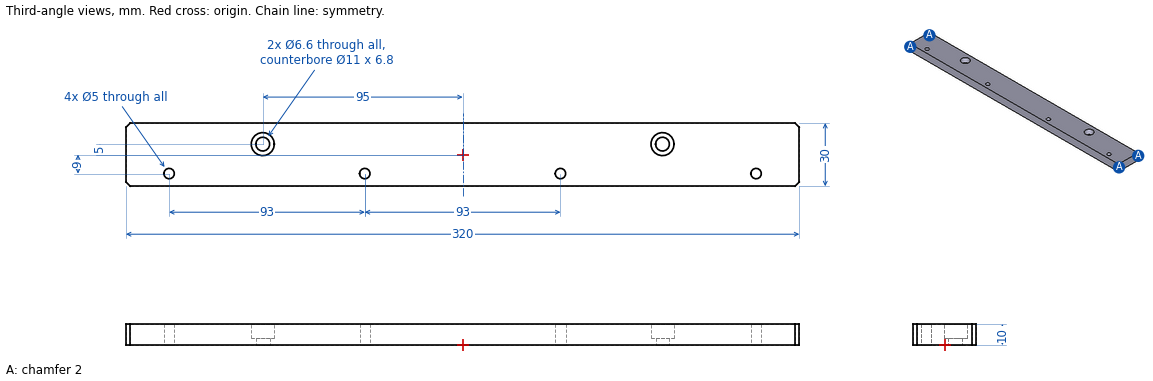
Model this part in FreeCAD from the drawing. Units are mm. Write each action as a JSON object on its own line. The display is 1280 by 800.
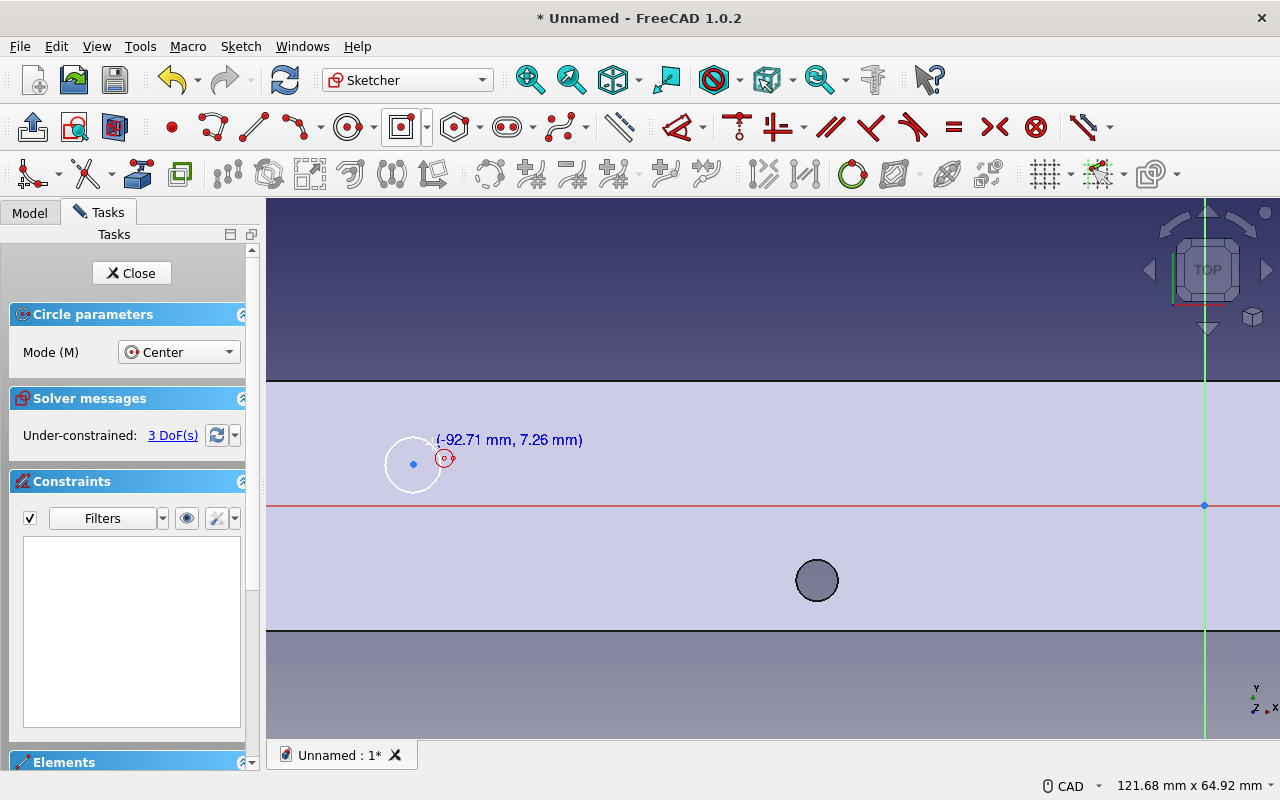
{"action": "scroll", "coordinate": [413, 467], "scroll_direction": "down", "scroll_amount": 5}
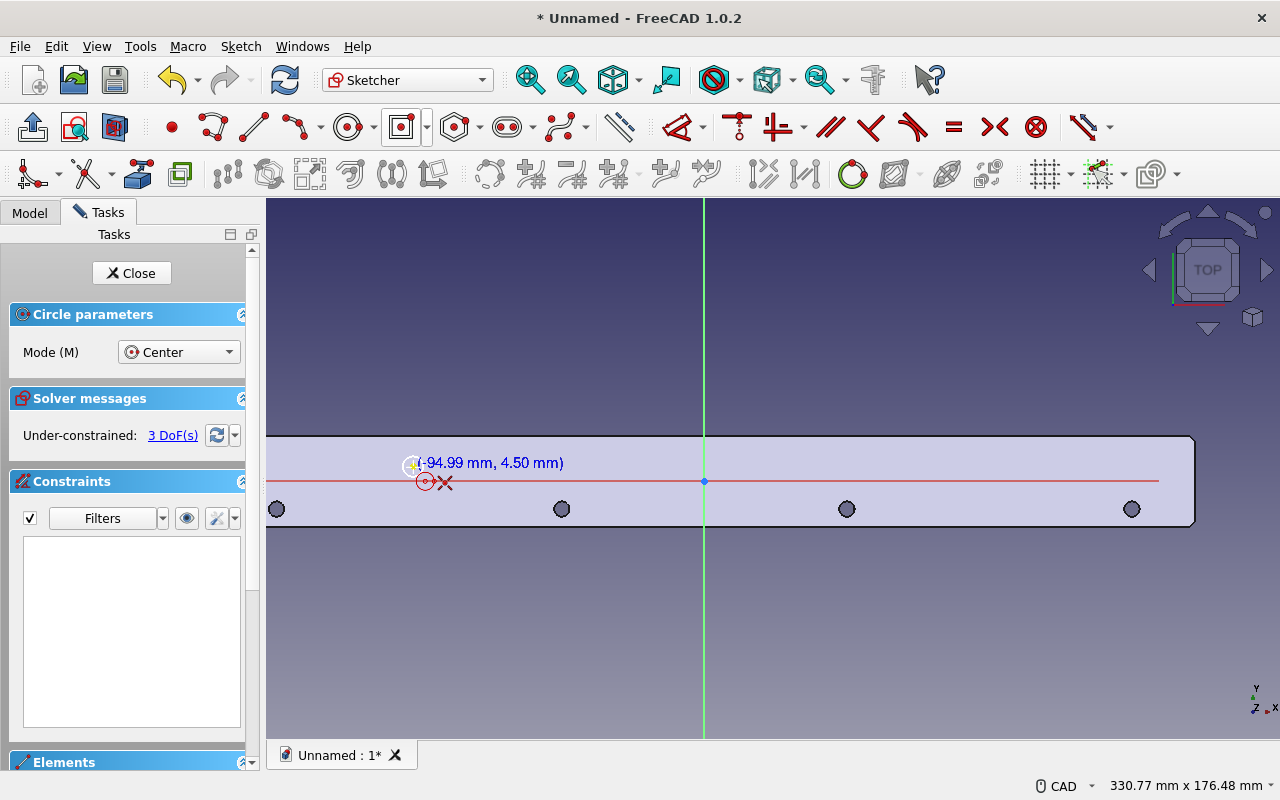
{"action": "scroll", "coordinate": [996, 466], "scroll_direction": "up", "scroll_amount": 5}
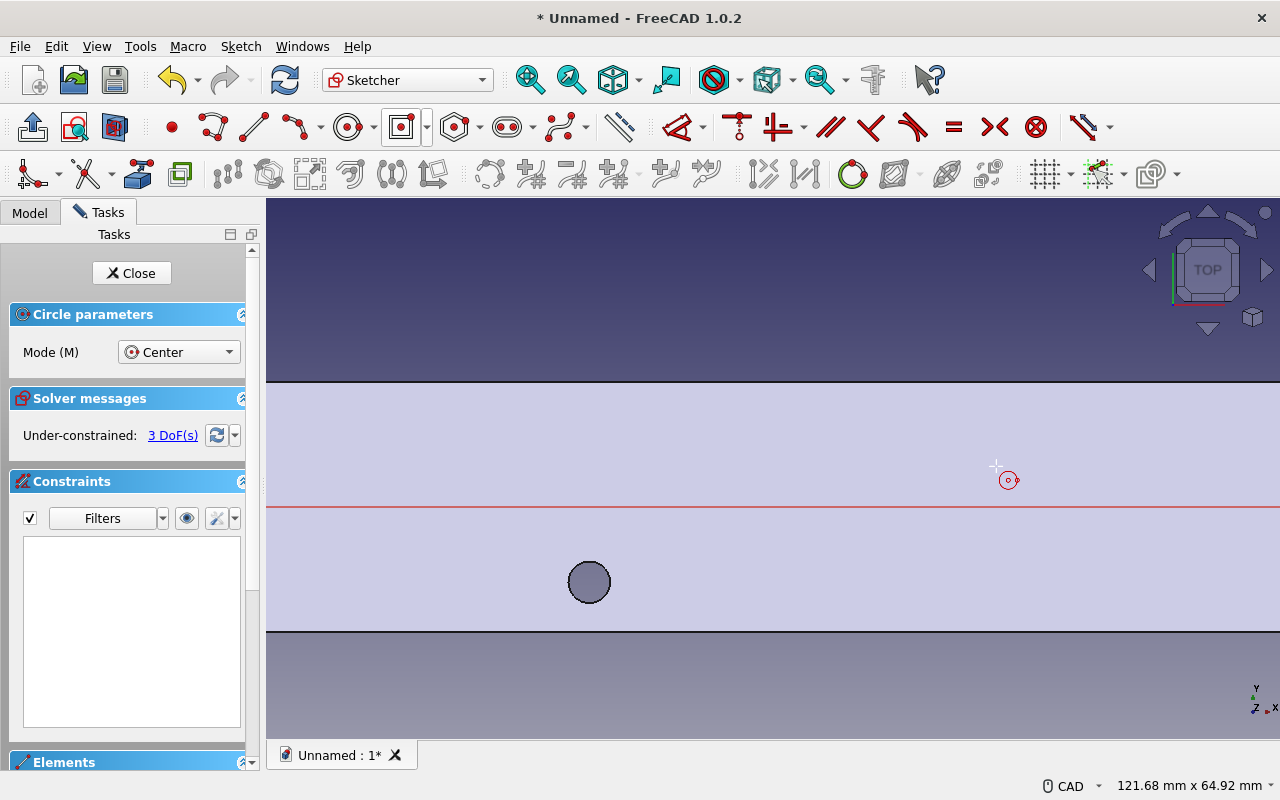
{"action": "left_click", "coordinate": [993, 466]}
{"action": "left_click", "coordinate": [1013, 446]}
{"action": "key", "text": "Escape"}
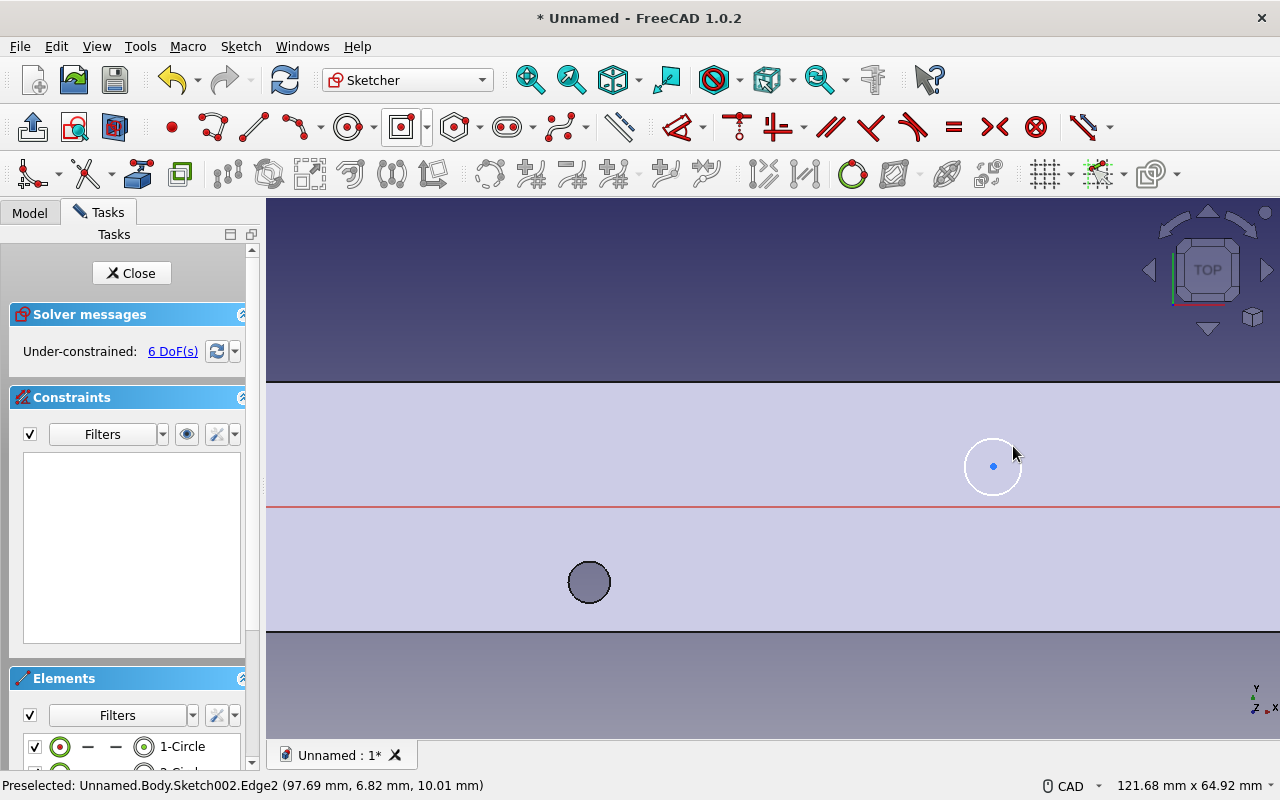
{"action": "scroll", "coordinate": [997, 466], "scroll_direction": "down", "scroll_amount": 5}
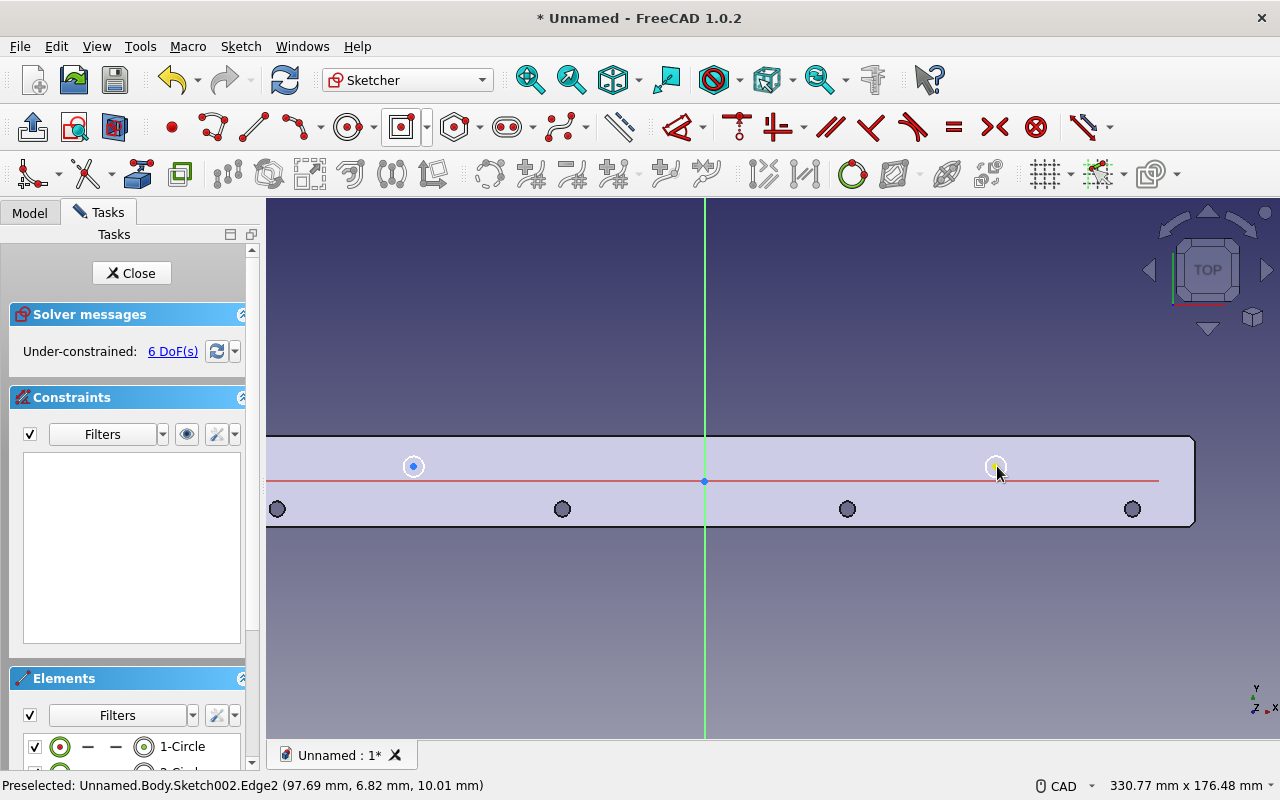
{"action": "scroll", "coordinate": [421, 459], "scroll_direction": "up", "scroll_amount": 2}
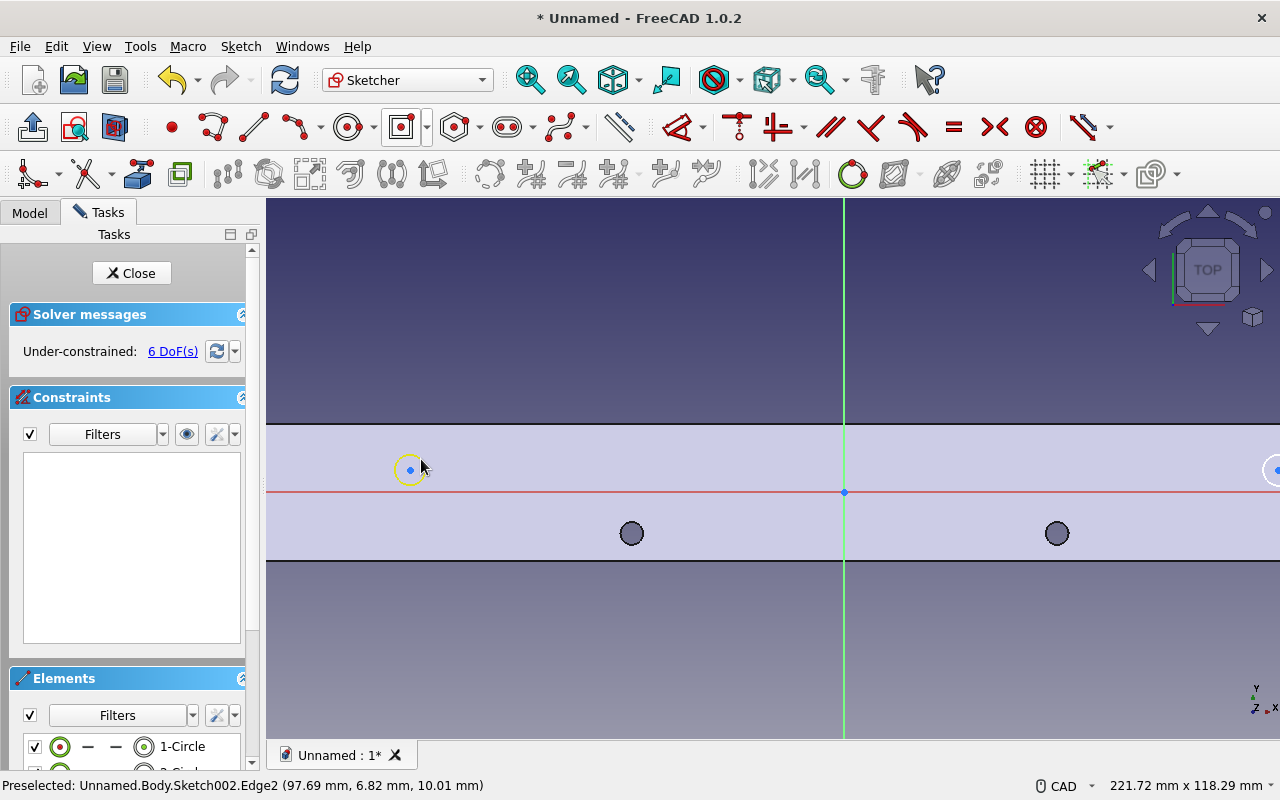
{"action": "left_click", "coordinate": [421, 459]}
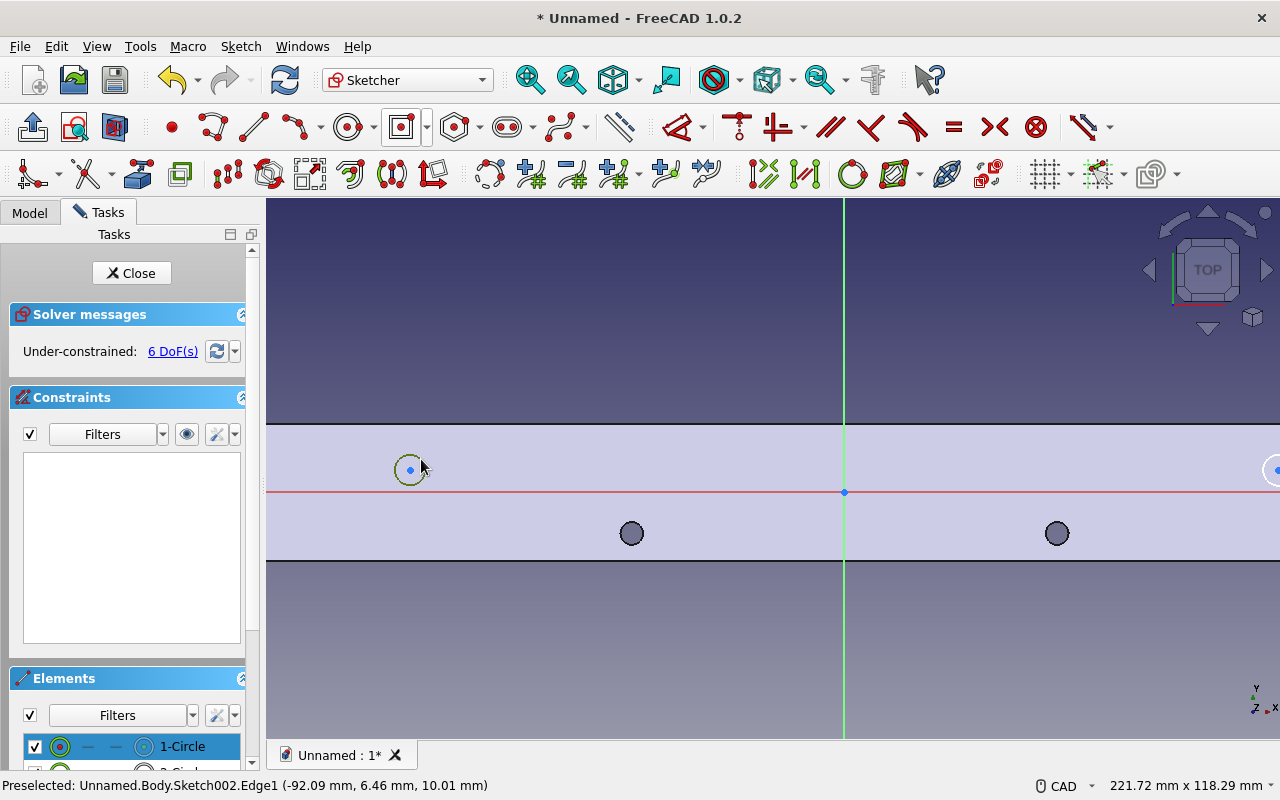
{"action": "scroll", "coordinate": [420, 459], "scroll_direction": "down", "scroll_amount": 2}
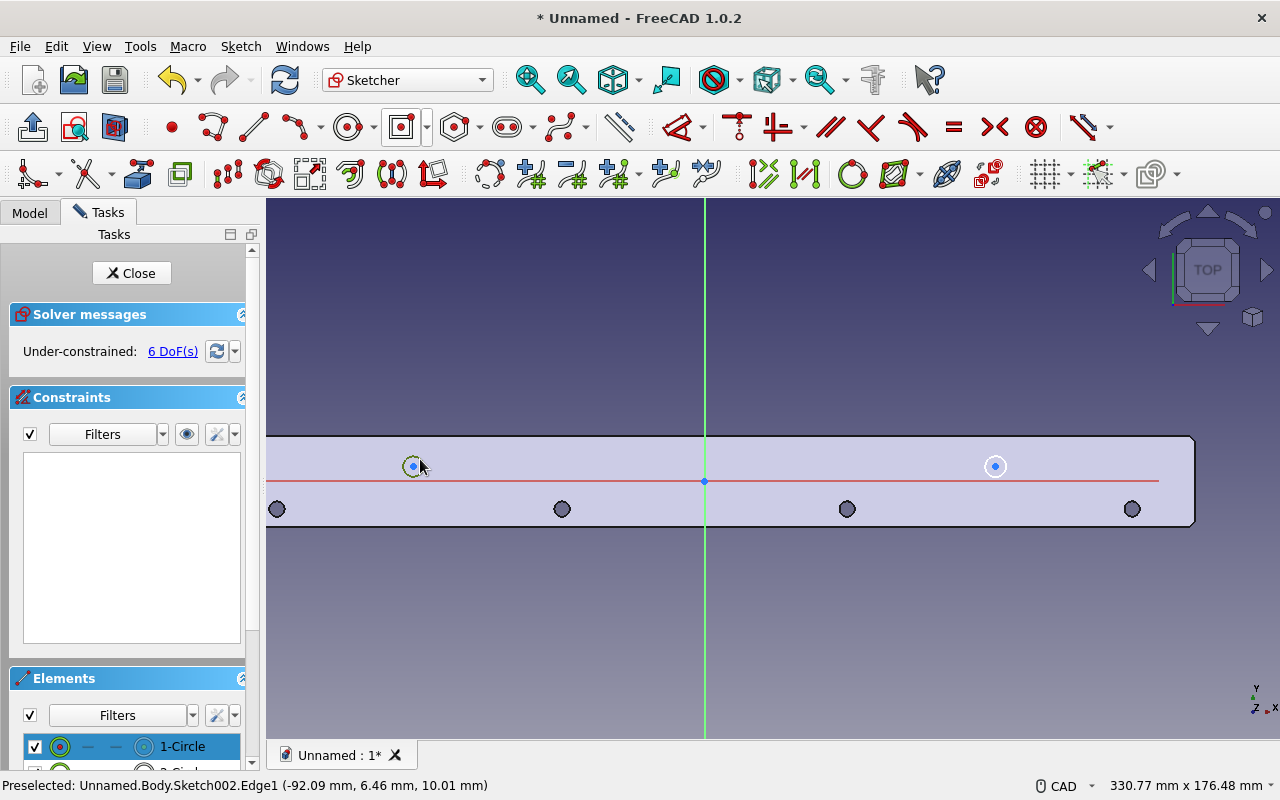
{"action": "scroll", "coordinate": [1003, 459], "scroll_direction": "up", "scroll_amount": 2}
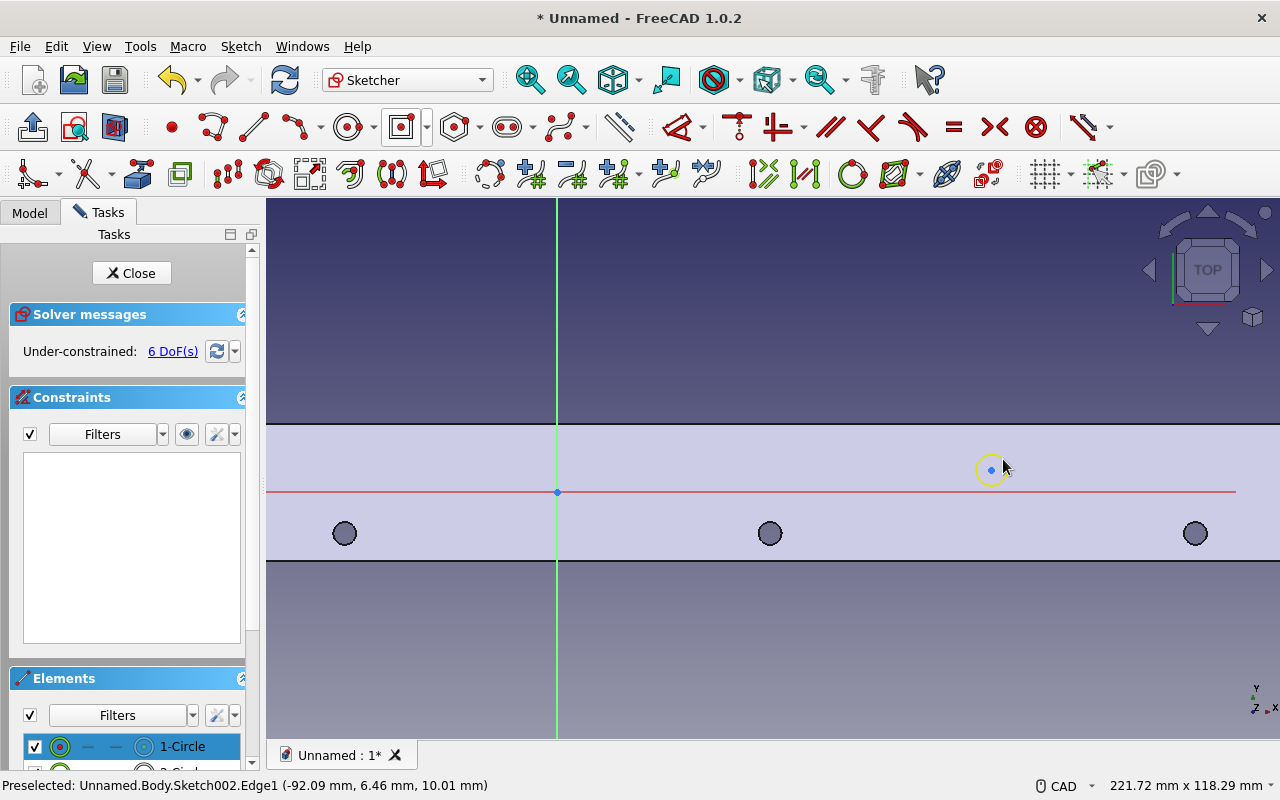
{"action": "left_click", "coordinate": [1003, 459]}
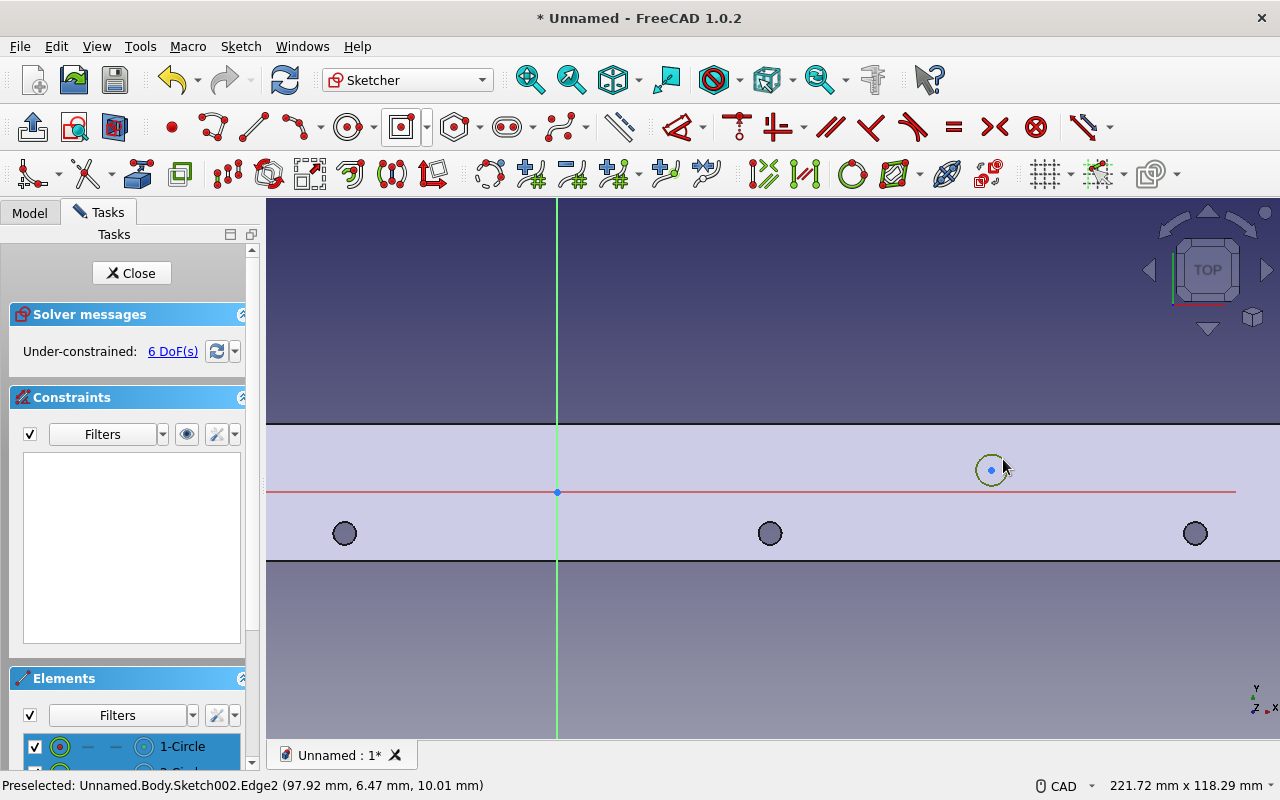
{"action": "left_click", "coordinate": [954, 128]}